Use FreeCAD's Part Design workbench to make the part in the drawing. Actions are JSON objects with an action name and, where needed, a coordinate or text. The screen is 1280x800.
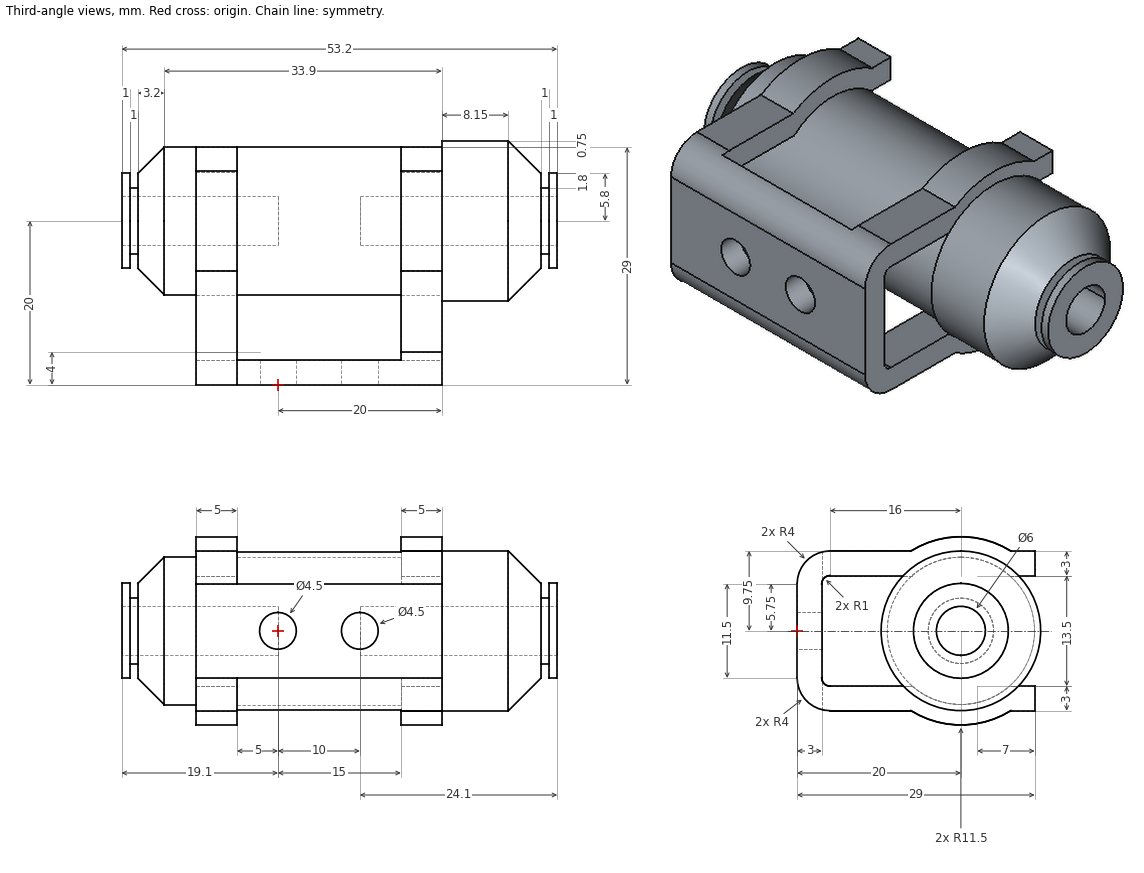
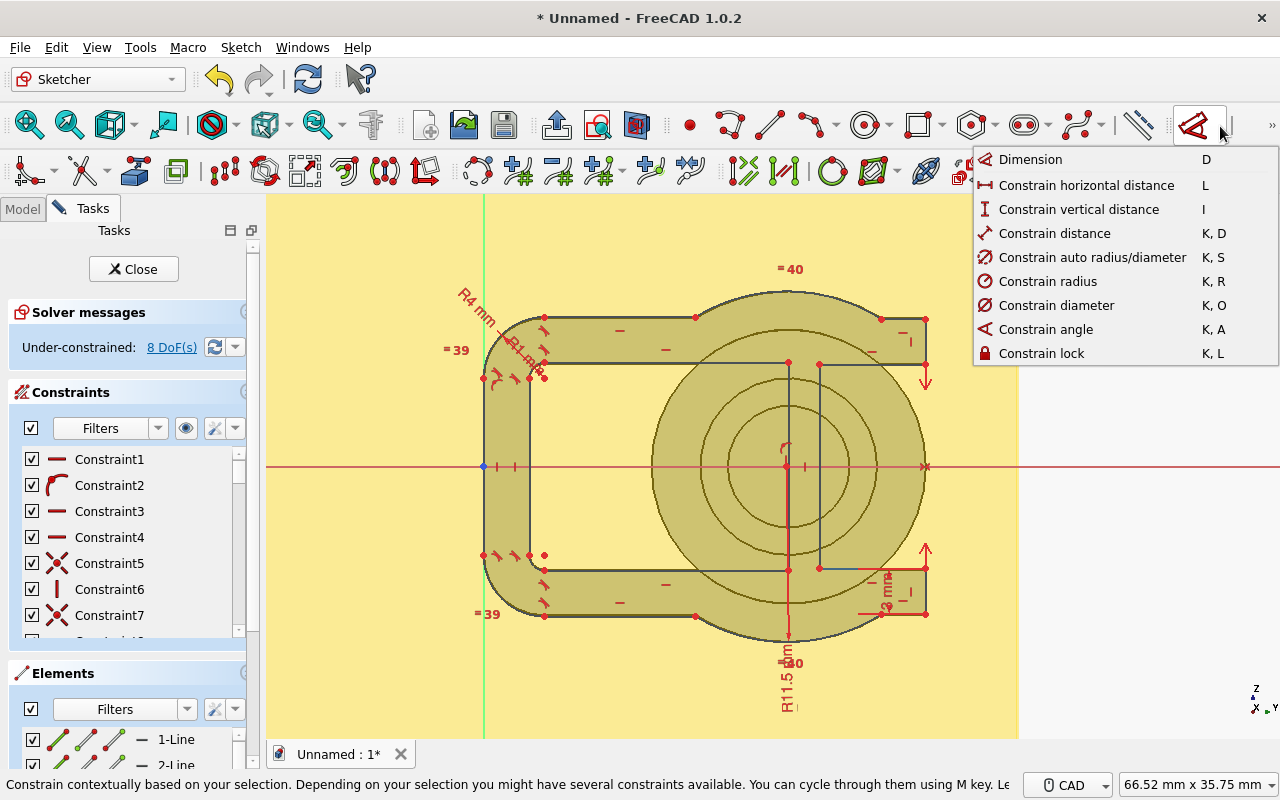
{"action": "left_click", "coordinate": [1126, 185]}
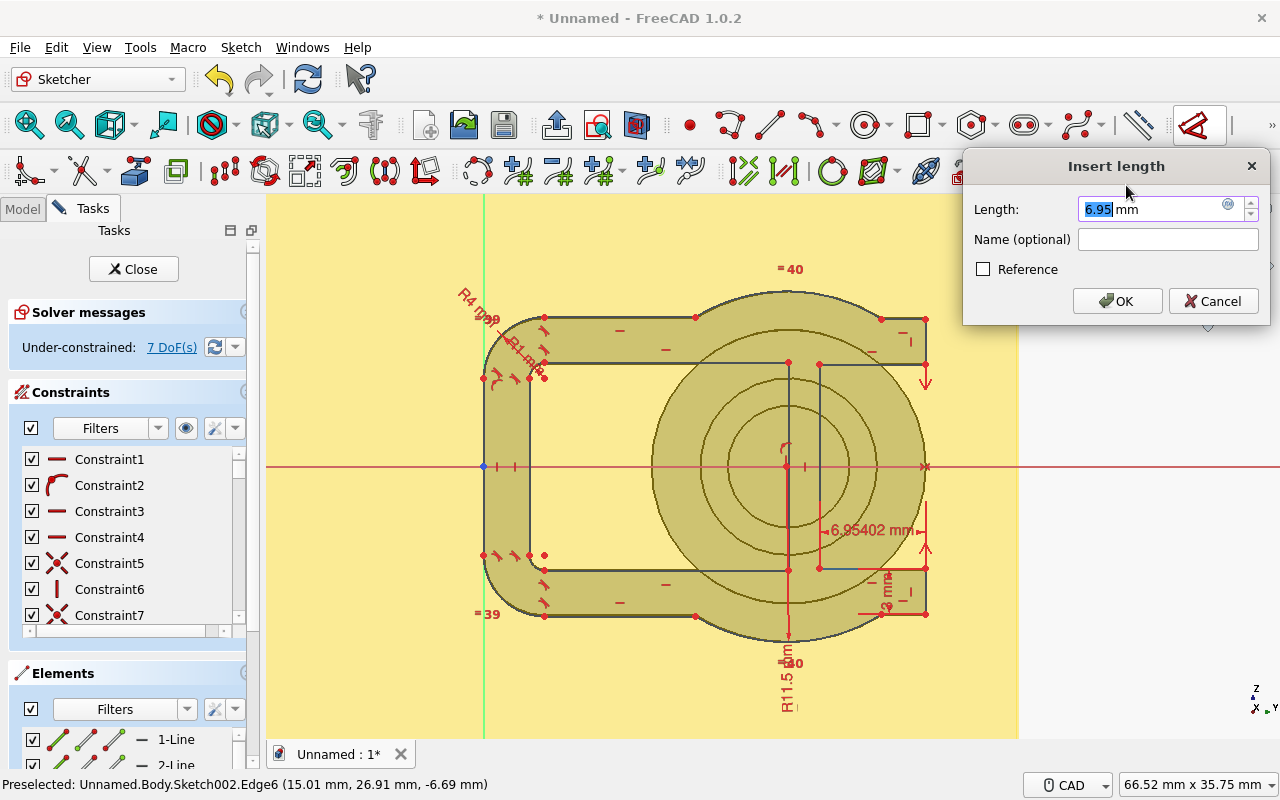
{"action": "type", "text": "7"}
{"action": "key", "text": "Return"}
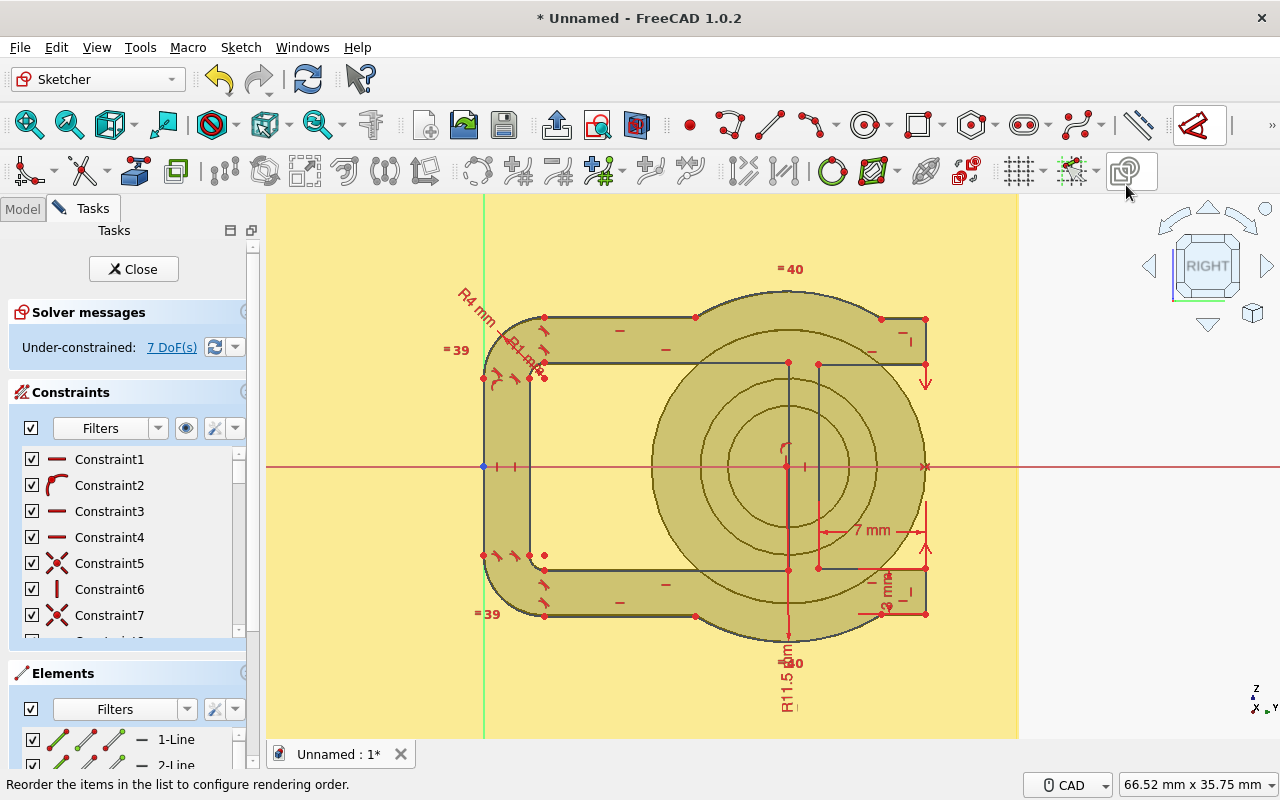
{"action": "left_click", "coordinate": [926, 351]}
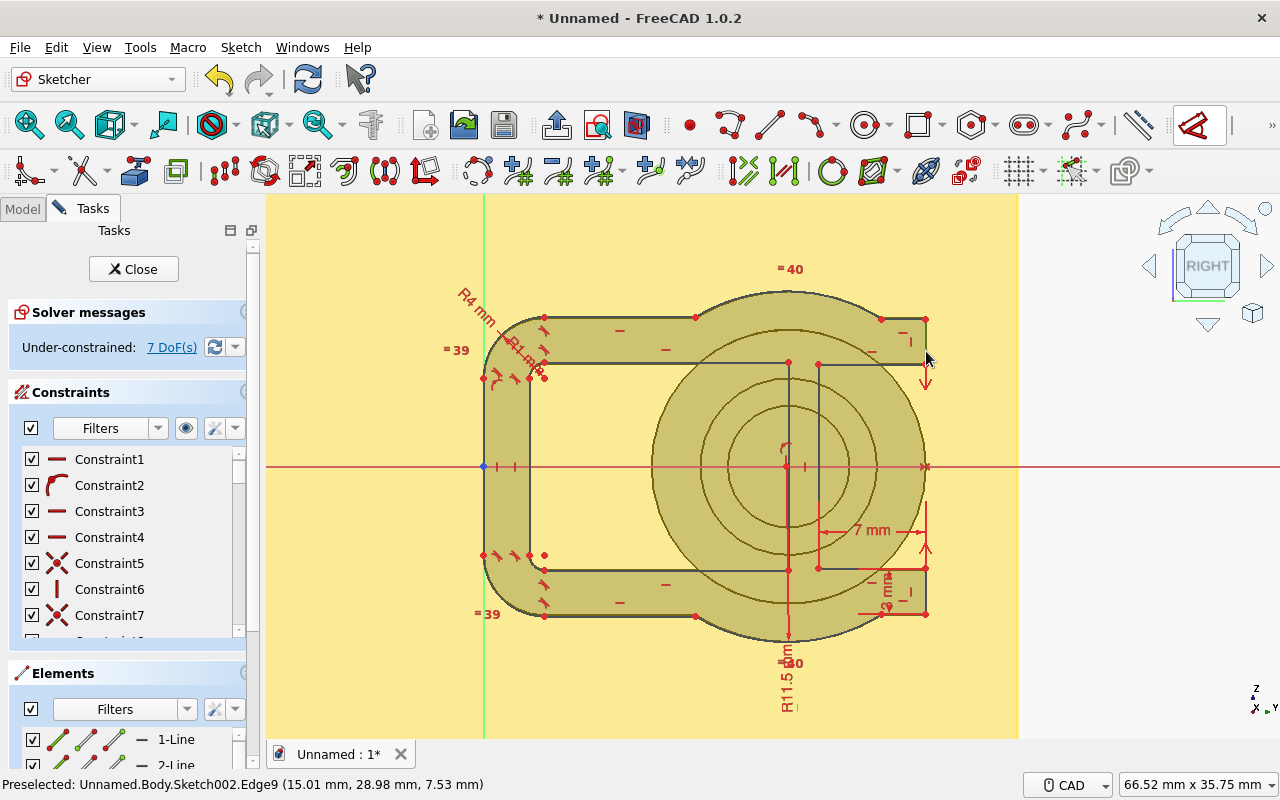
{"action": "left_click", "coordinate": [1220, 126]}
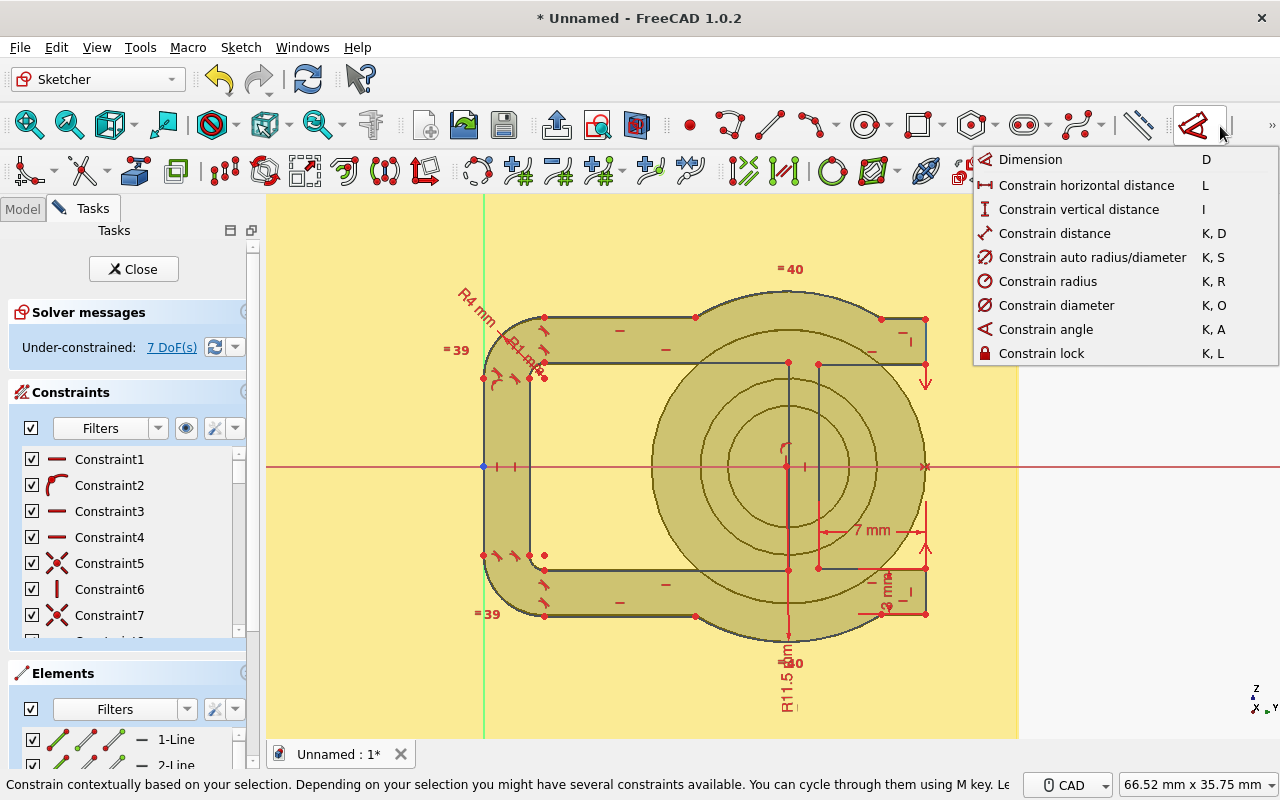
{"action": "left_click", "coordinate": [1126, 209]}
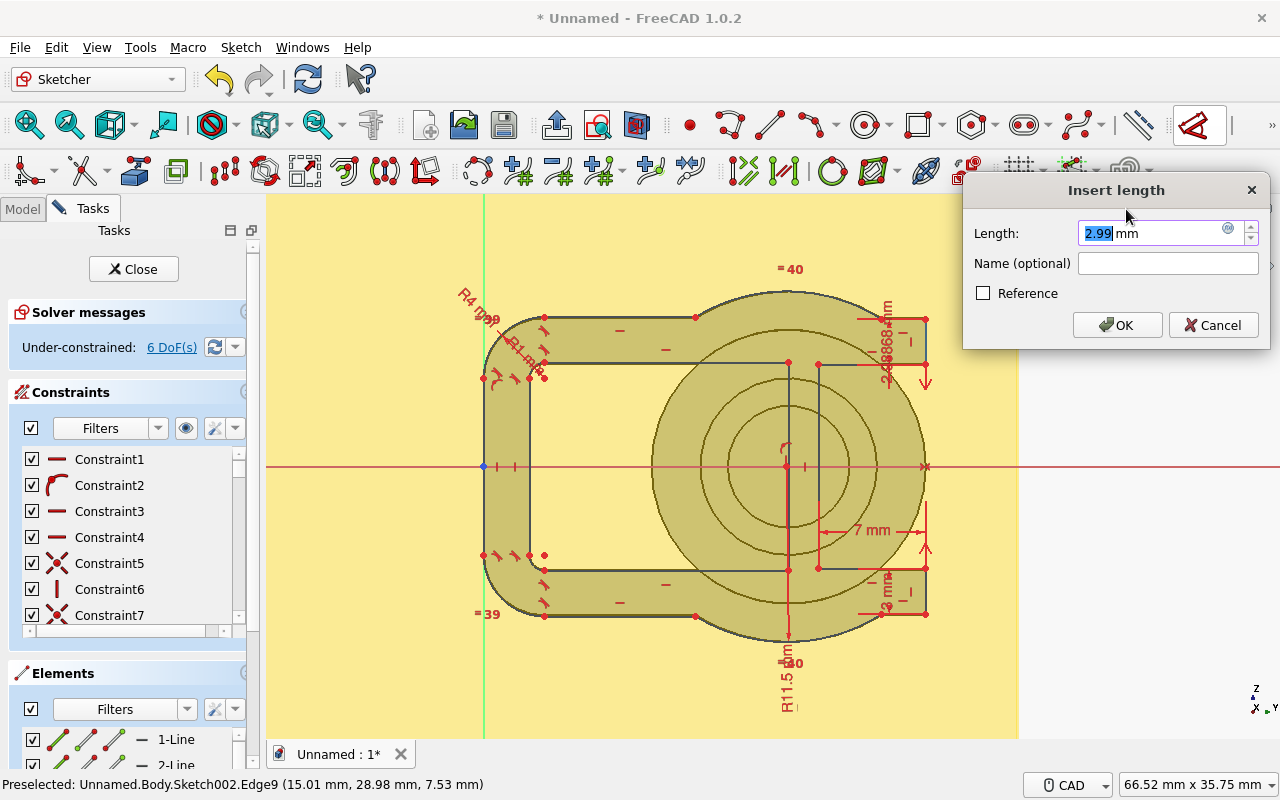
{"action": "type", "text": "3"}
{"action": "key", "text": "Return"}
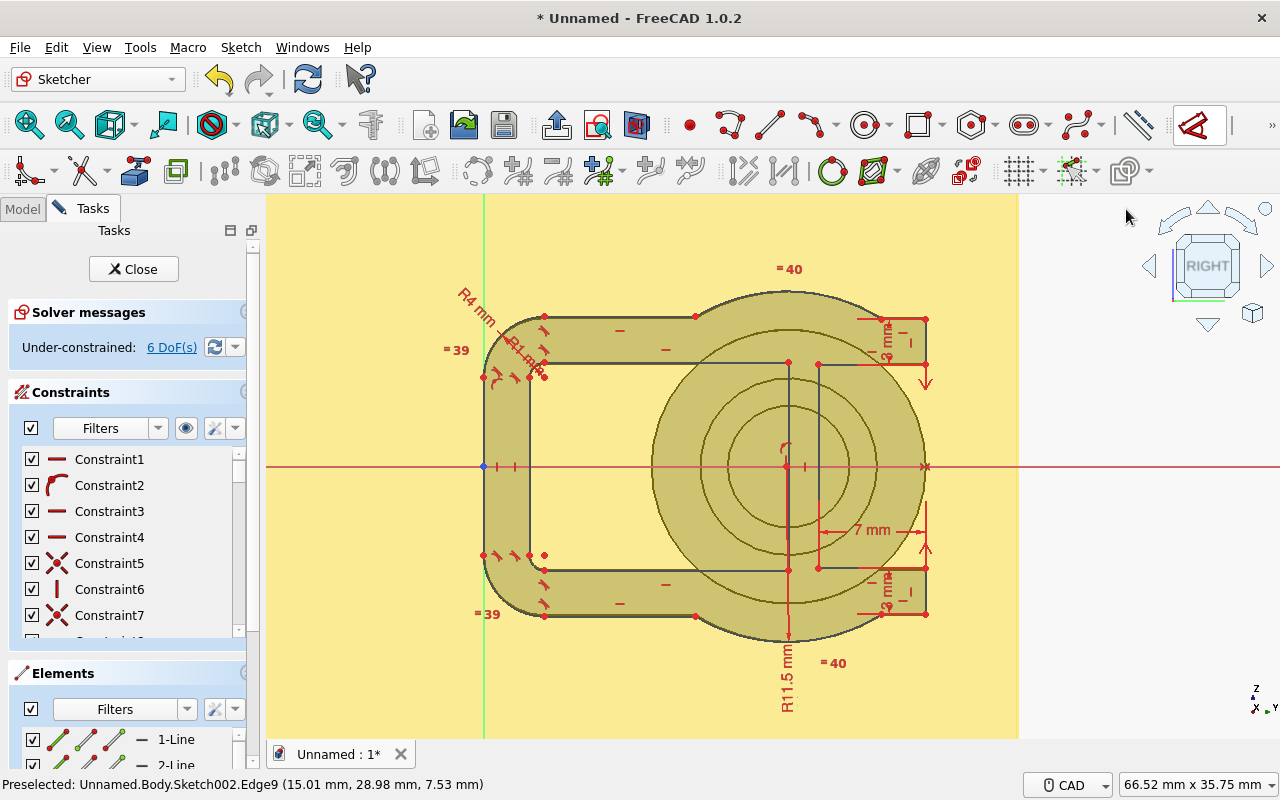
{"action": "left_click", "coordinate": [618, 363]}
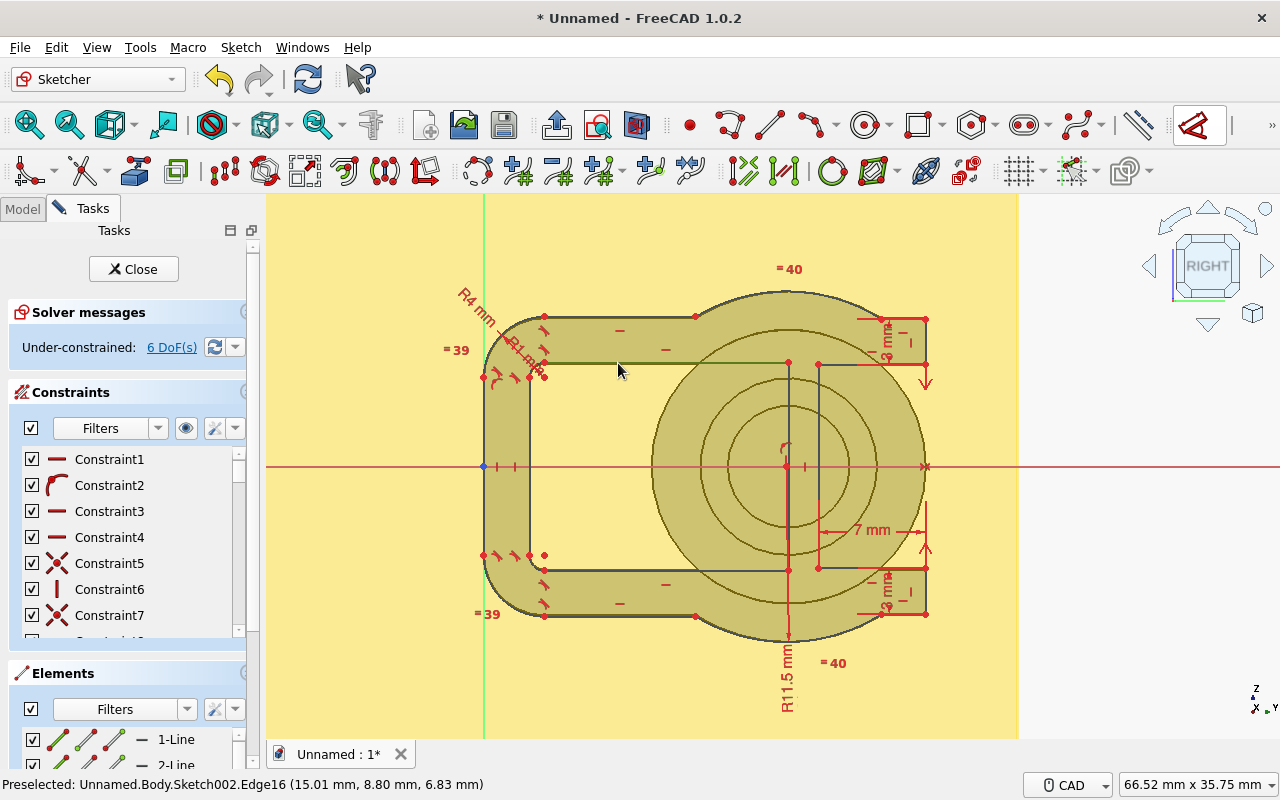
{"action": "left_click", "coordinate": [1220, 126]}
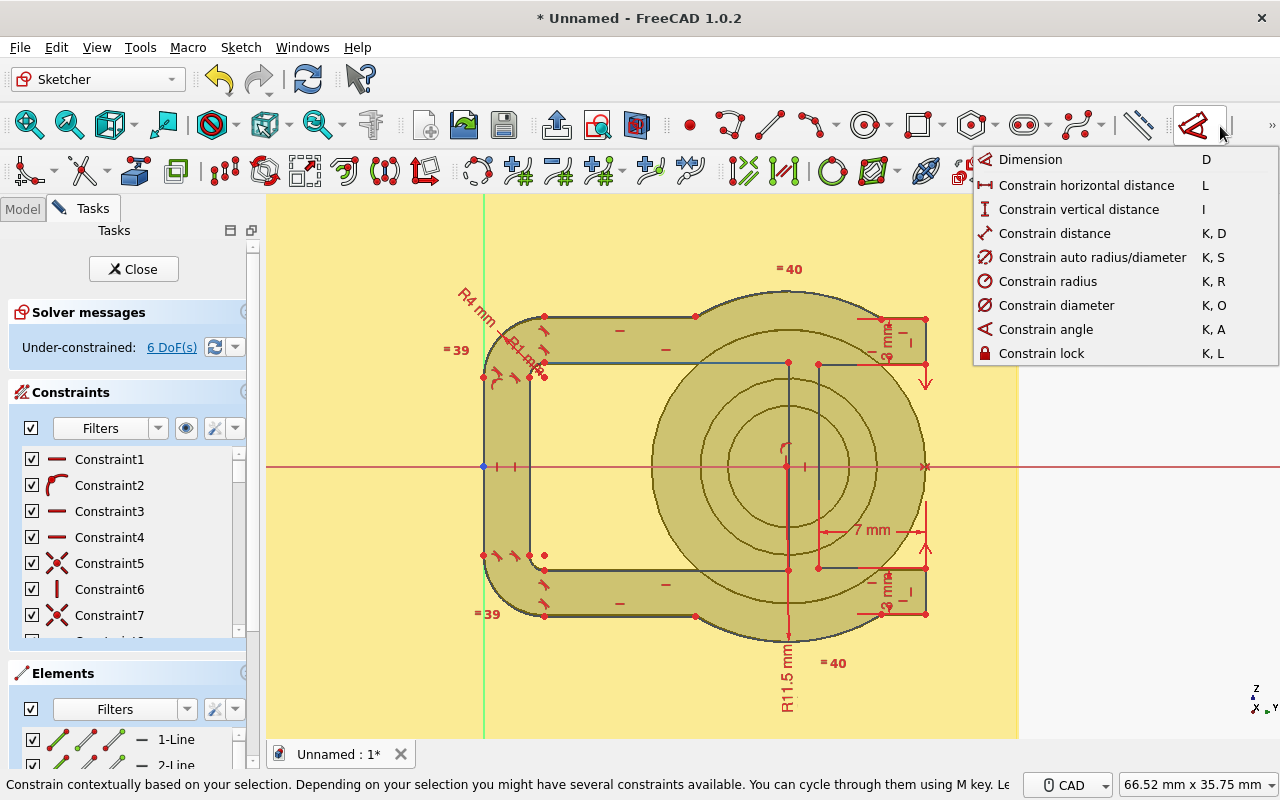
{"action": "left_click", "coordinate": [1126, 185]}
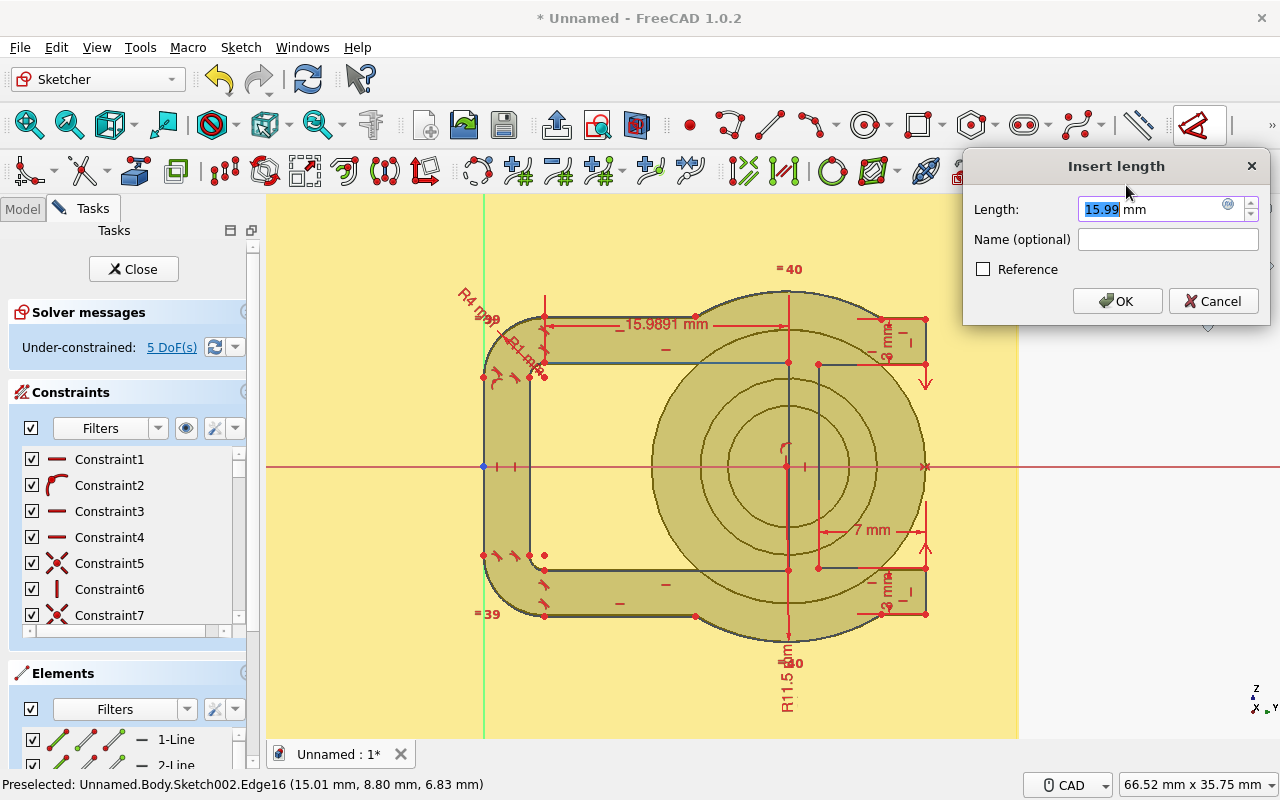
{"action": "type", "text": "16"}
{"action": "key", "text": "Return"}